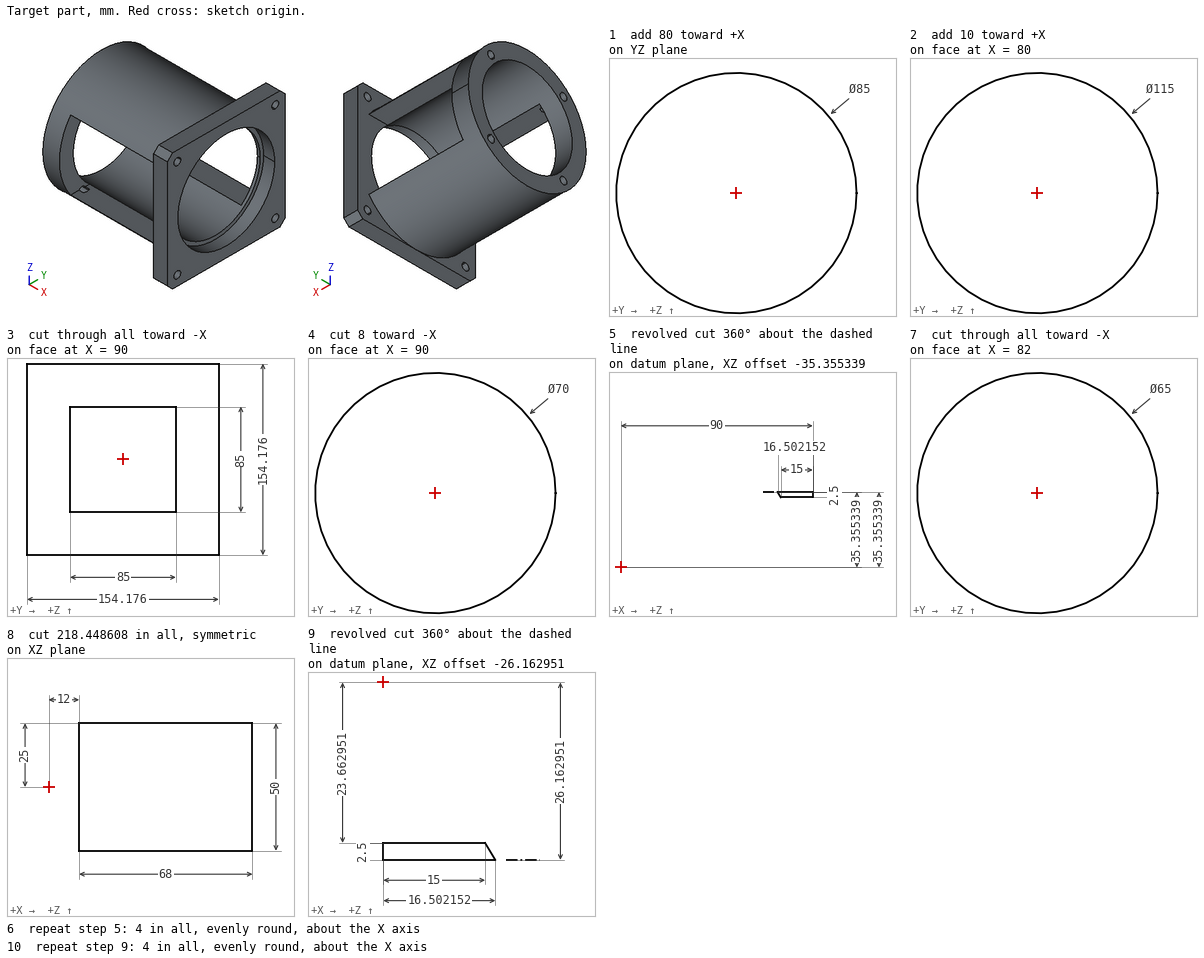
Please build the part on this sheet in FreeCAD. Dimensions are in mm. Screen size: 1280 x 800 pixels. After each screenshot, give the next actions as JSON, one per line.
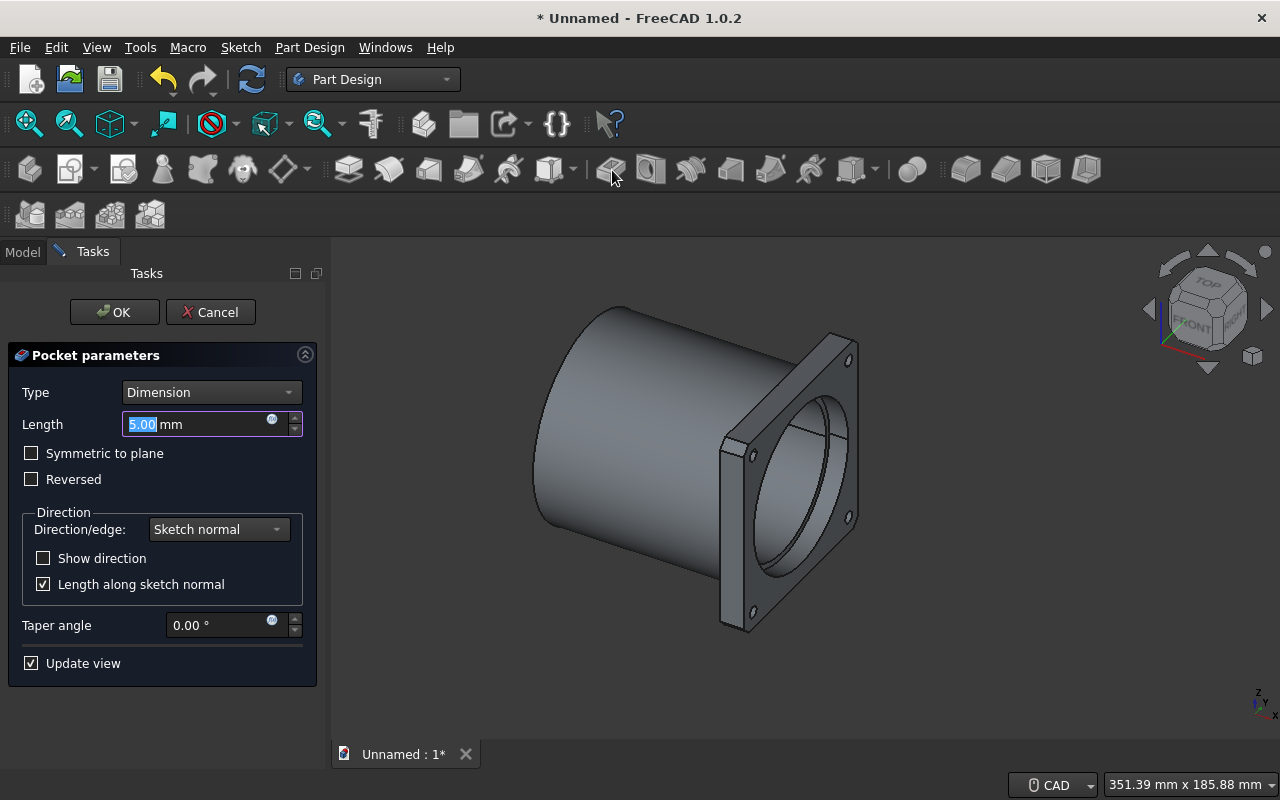
{"action": "type", "text": "218.448608"}
{"action": "key", "text": "Tab"}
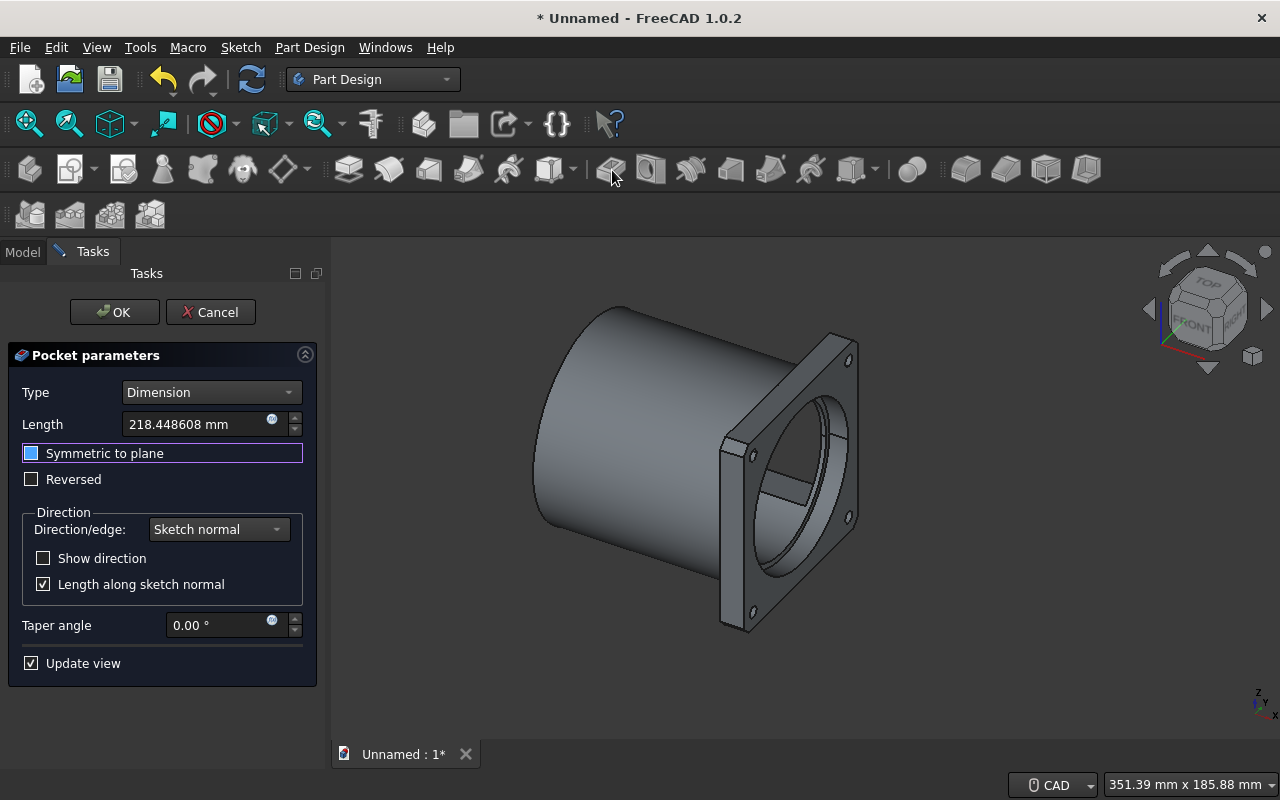
{"action": "left_click", "coordinate": [30, 453]}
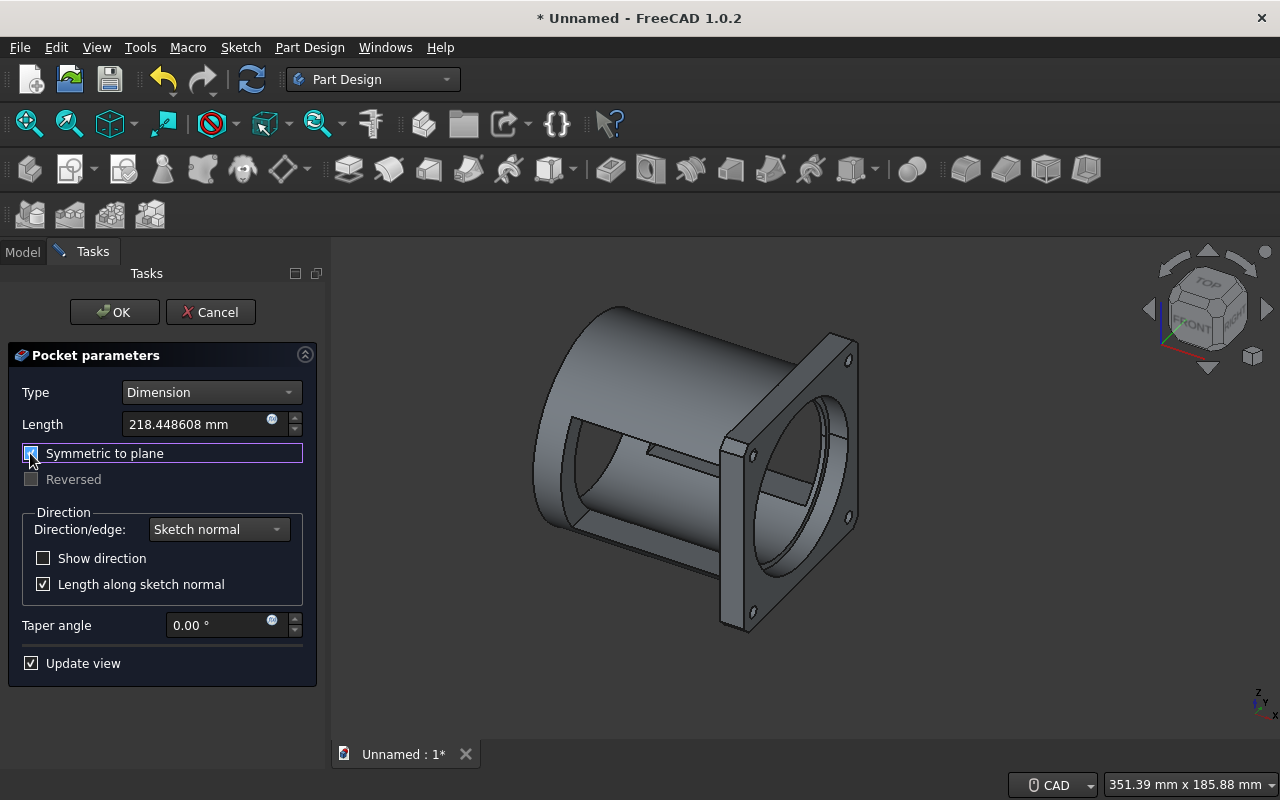
{"action": "left_click", "coordinate": [115, 312]}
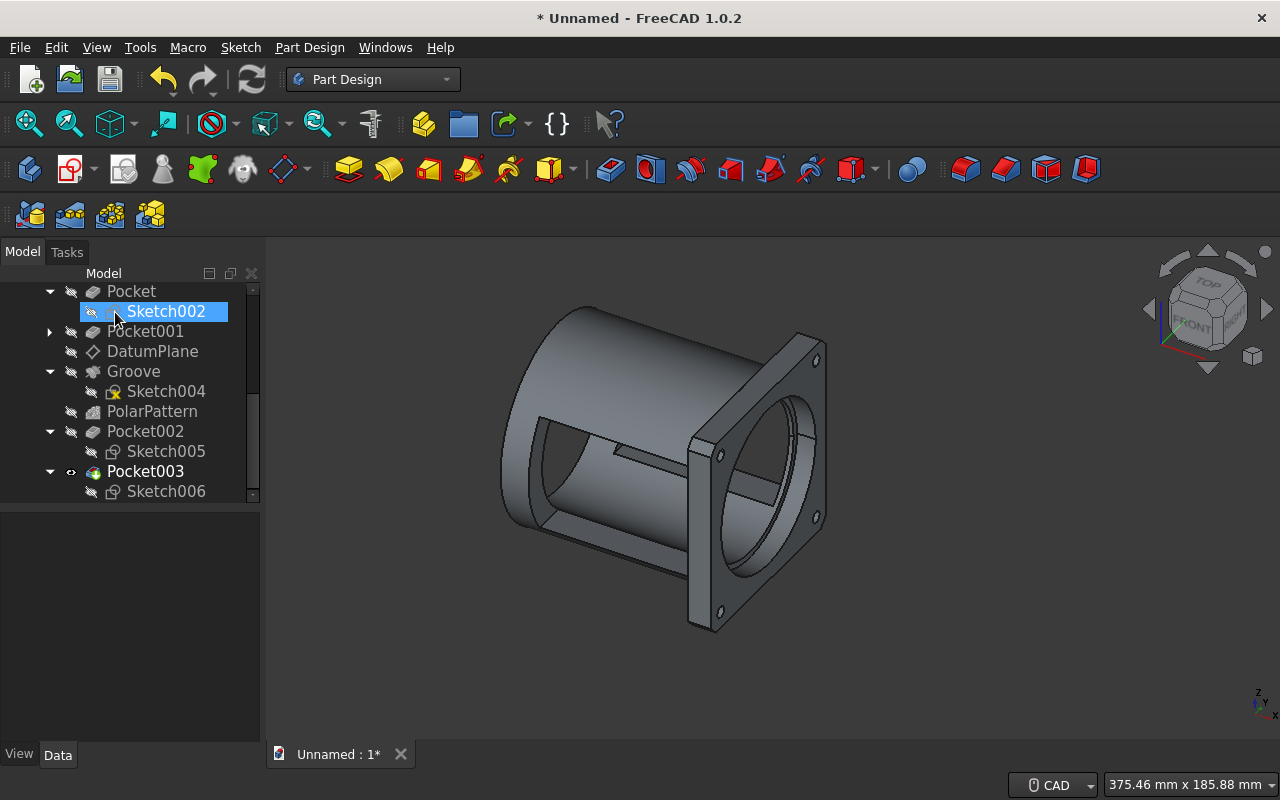
{"action": "scroll", "coordinate": [140, 387], "scroll_direction": "down", "scroll_amount": 3}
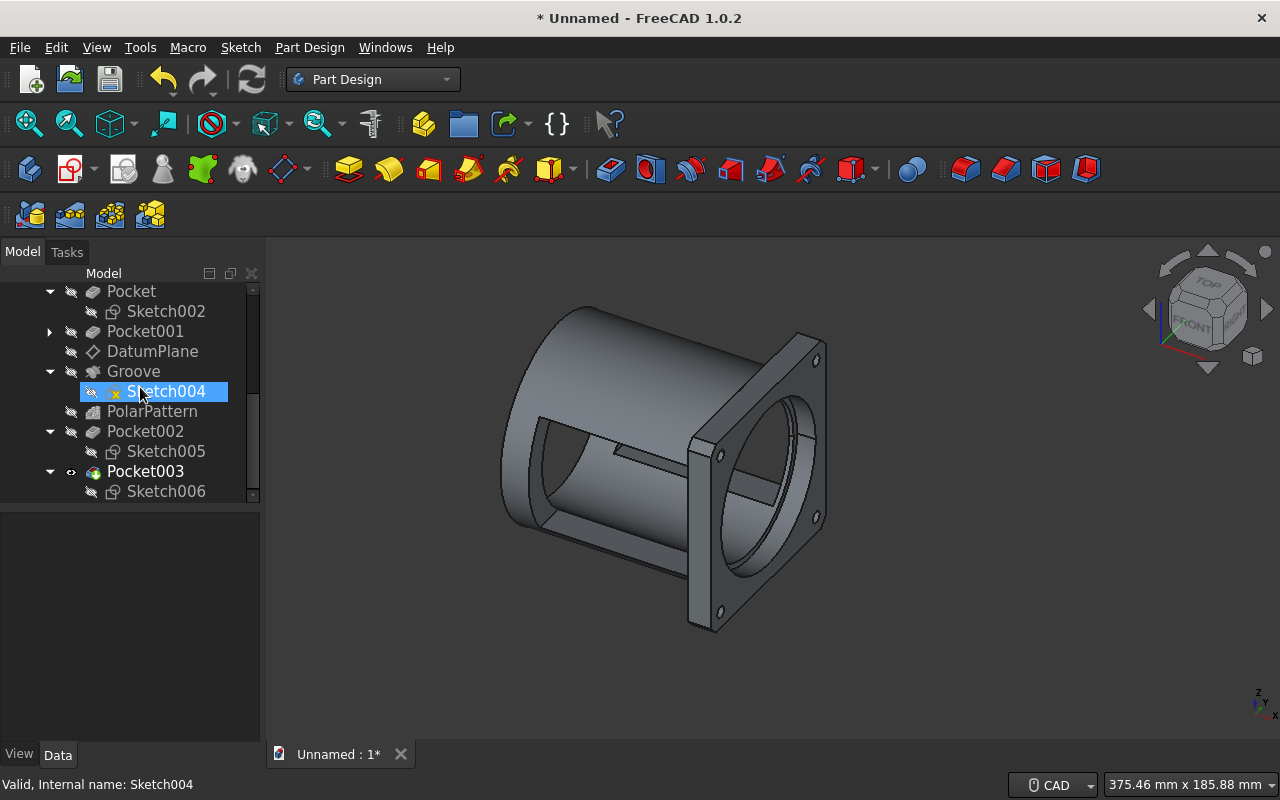
{"action": "scroll", "coordinate": [140, 387], "scroll_direction": "up", "scroll_amount": 15}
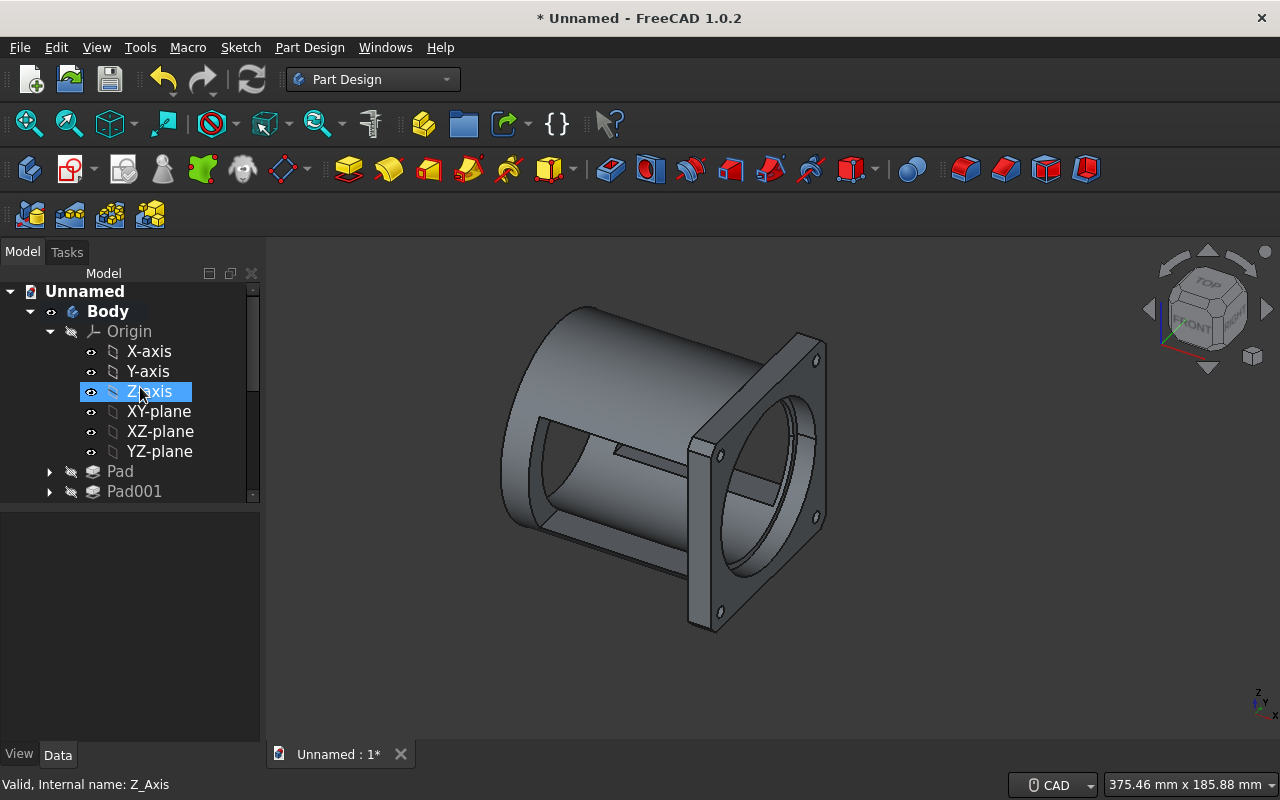
{"action": "left_click", "coordinate": [136, 432]}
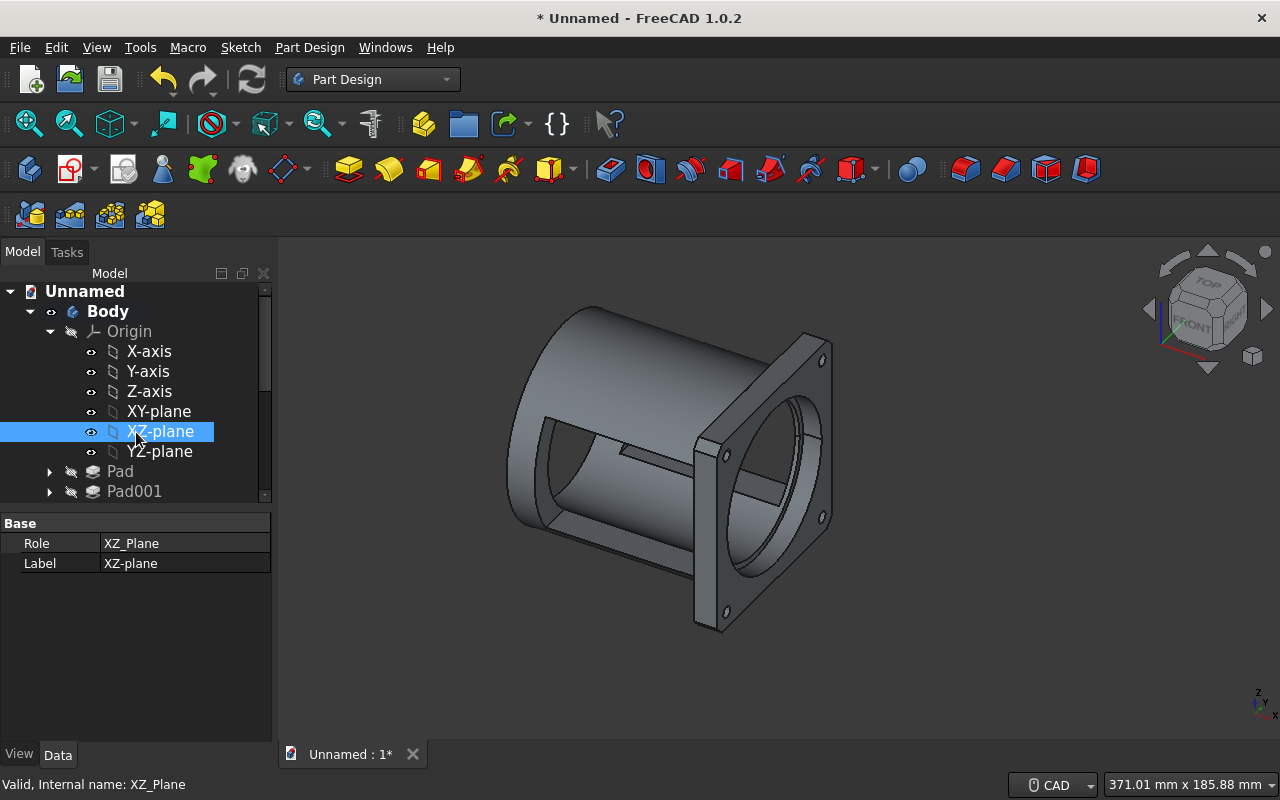
{"action": "left_click", "coordinate": [284, 170]}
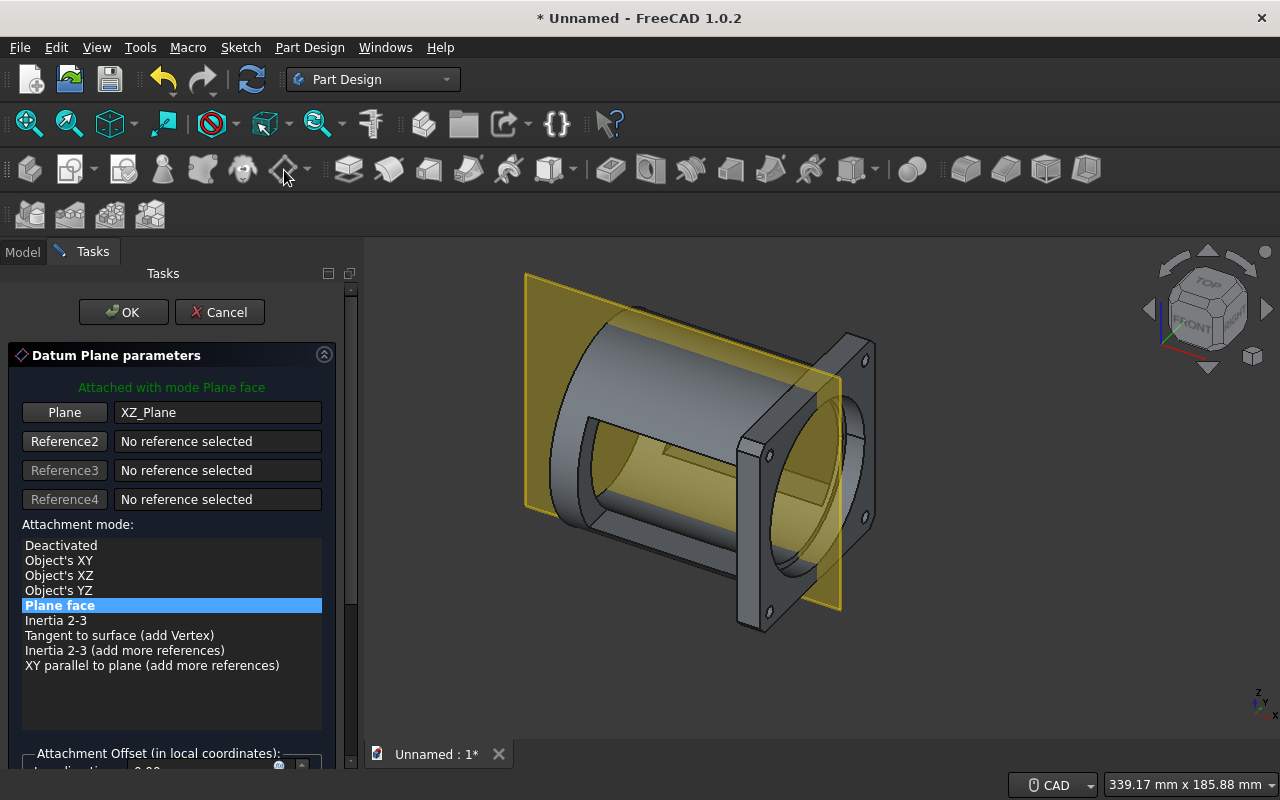
{"action": "scroll", "coordinate": [351, 526], "scroll_direction": "down", "scroll_amount": 3}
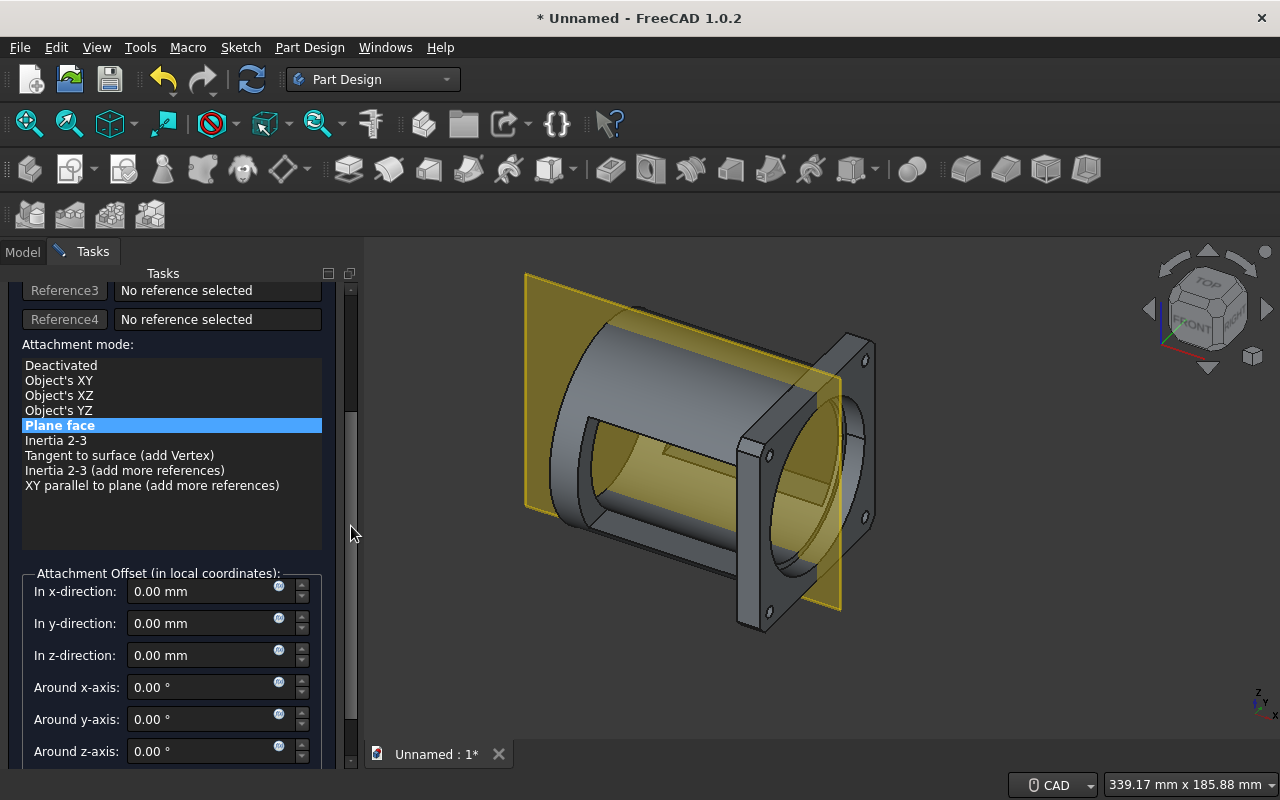
{"action": "triple_click", "coordinate": [210, 655]}